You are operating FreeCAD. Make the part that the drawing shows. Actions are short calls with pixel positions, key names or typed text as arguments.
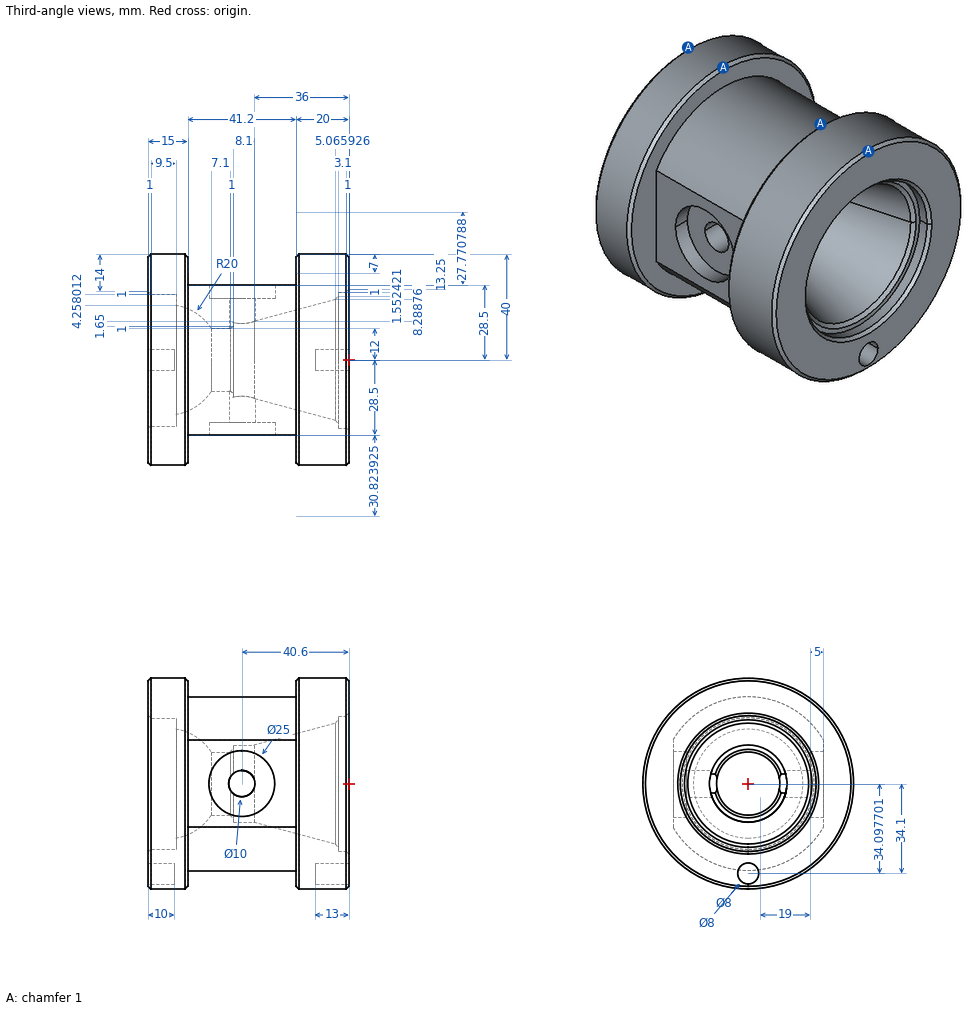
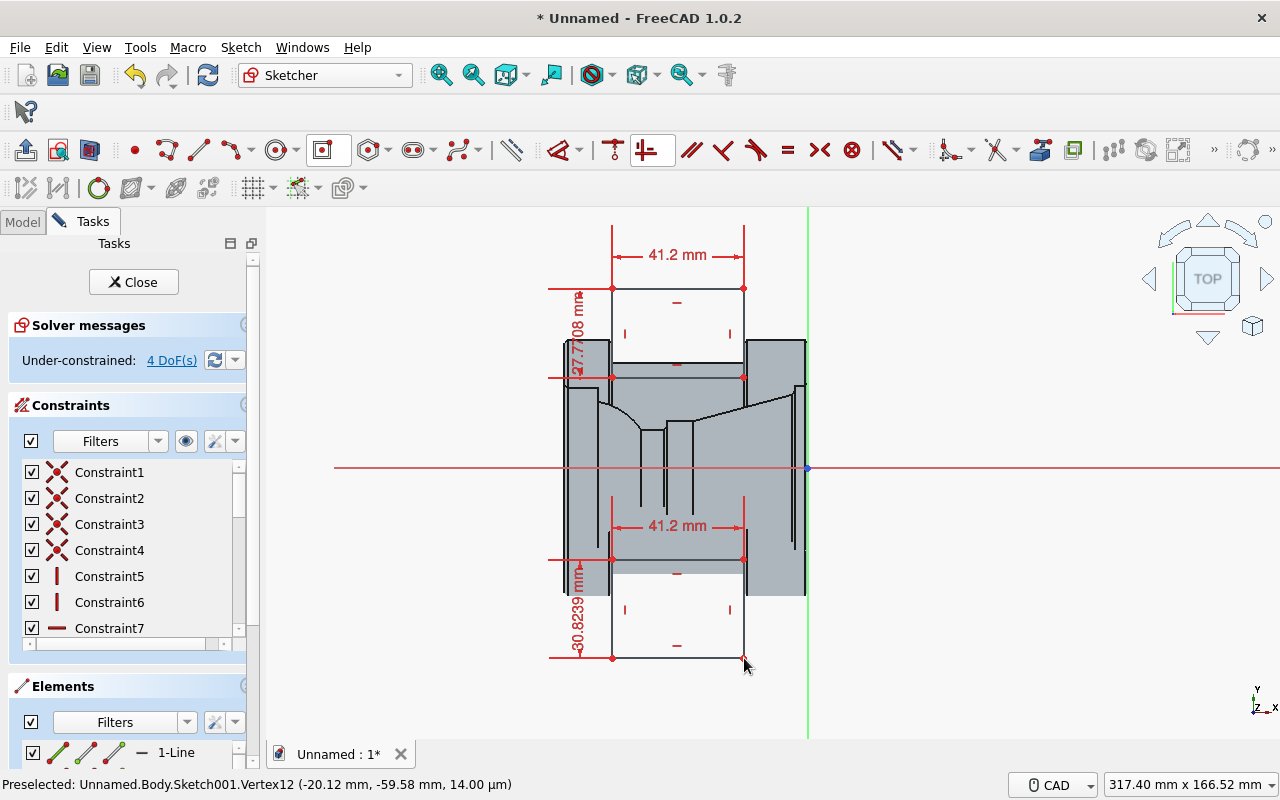
click(558, 150)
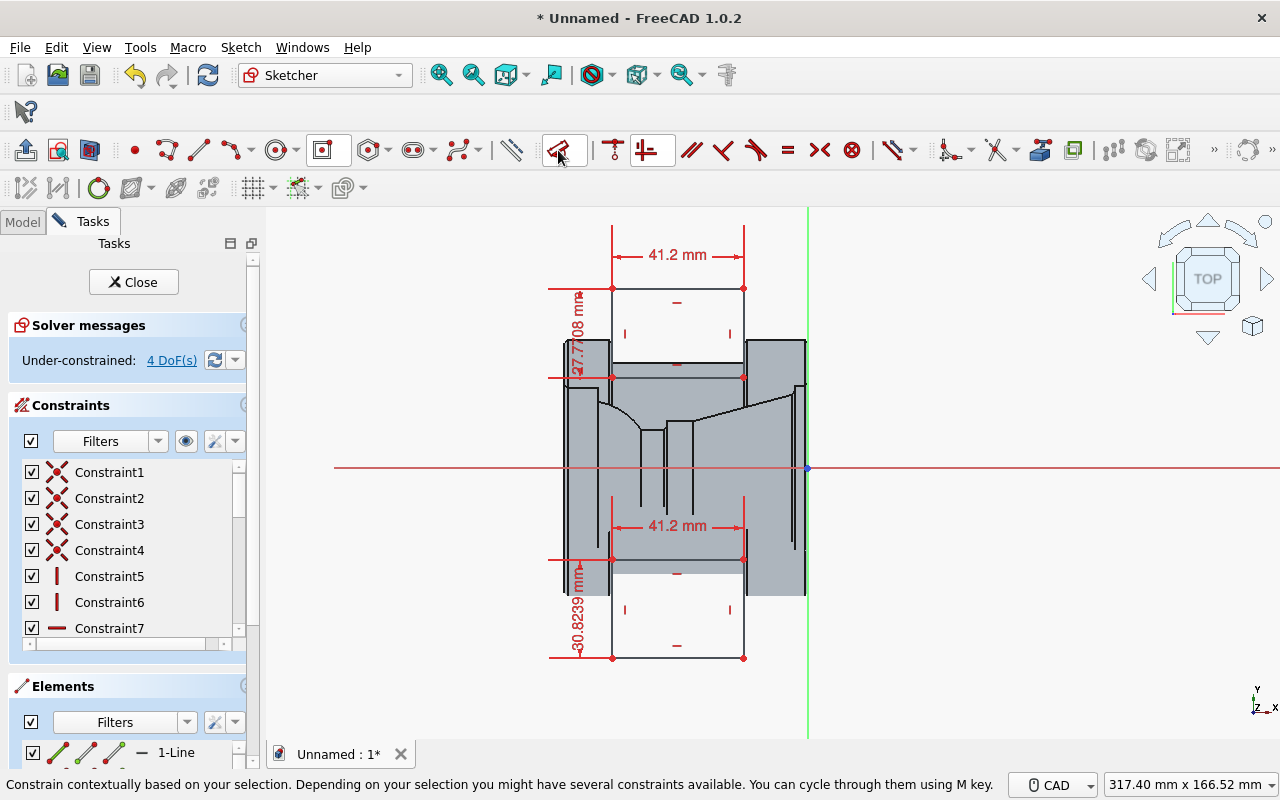
click(744, 378)
click(776, 344)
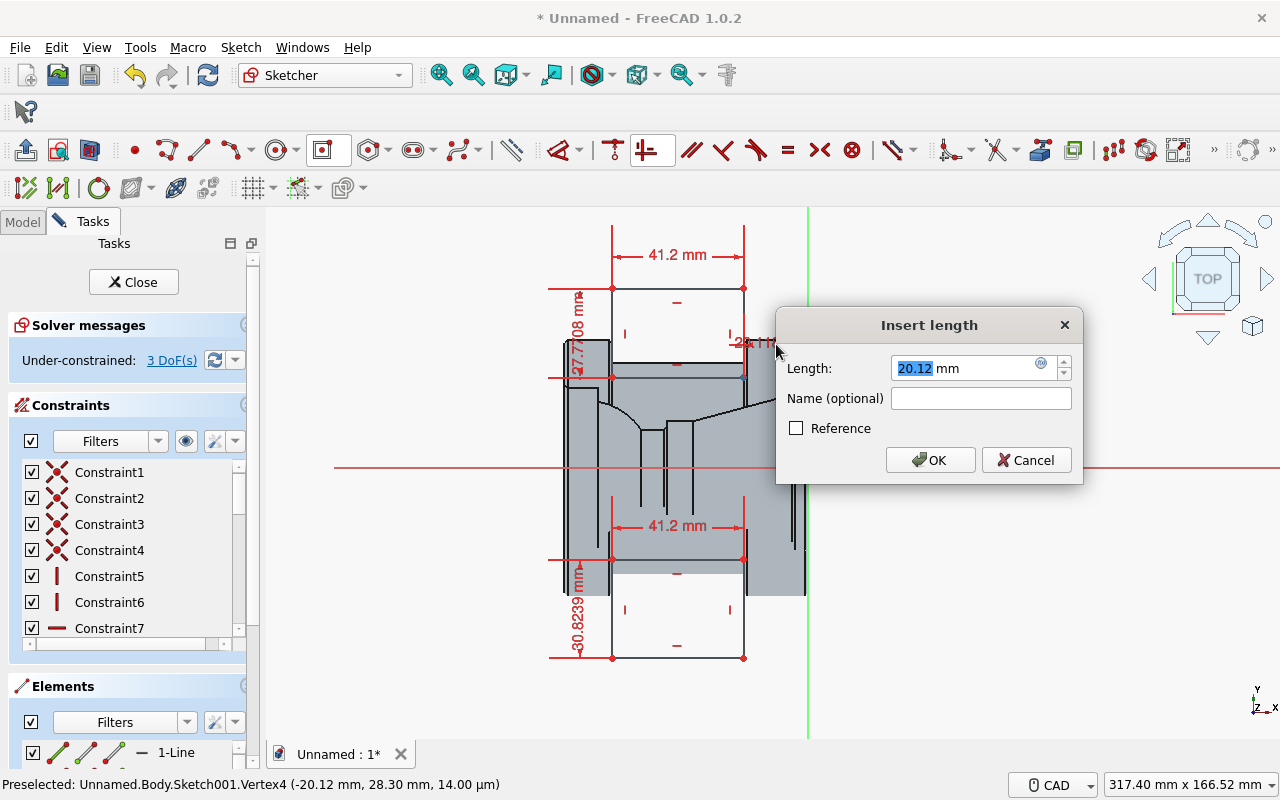
text(20)
key(Return)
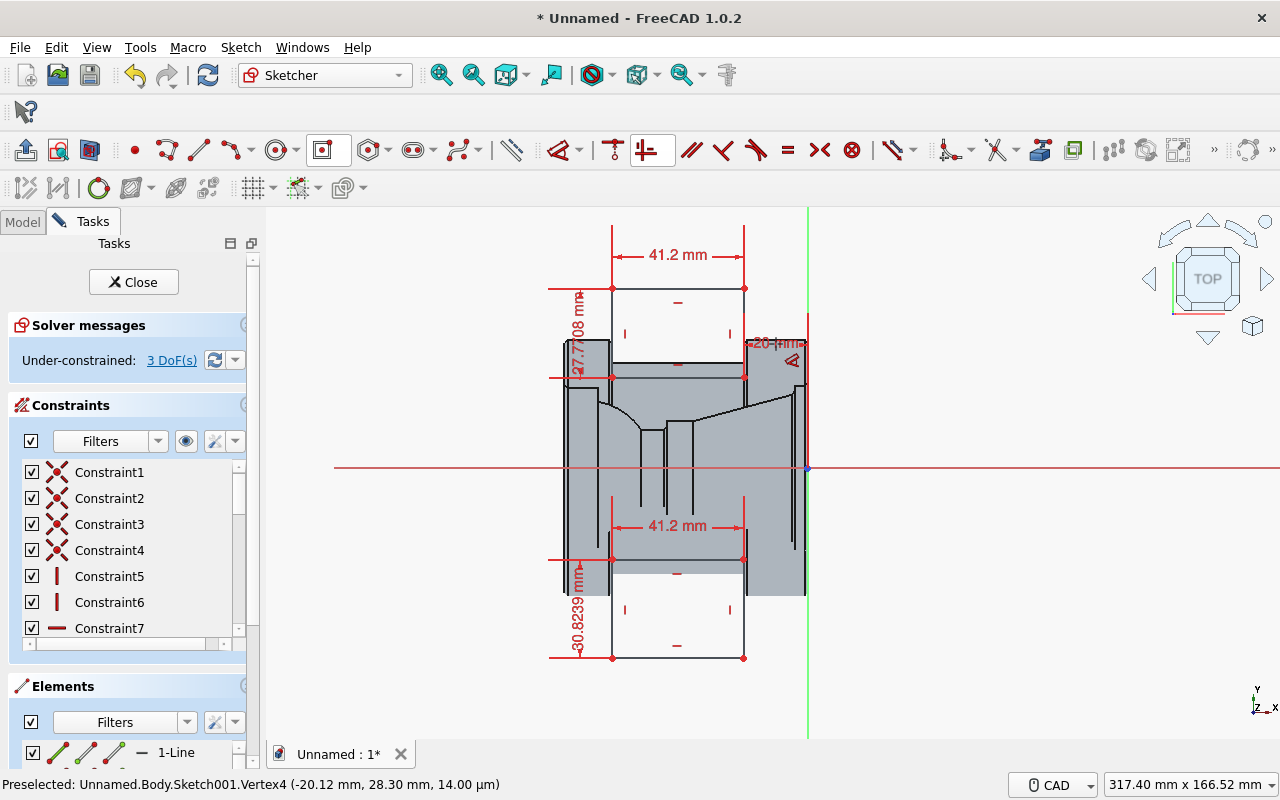
click(744, 658)
click(776, 692)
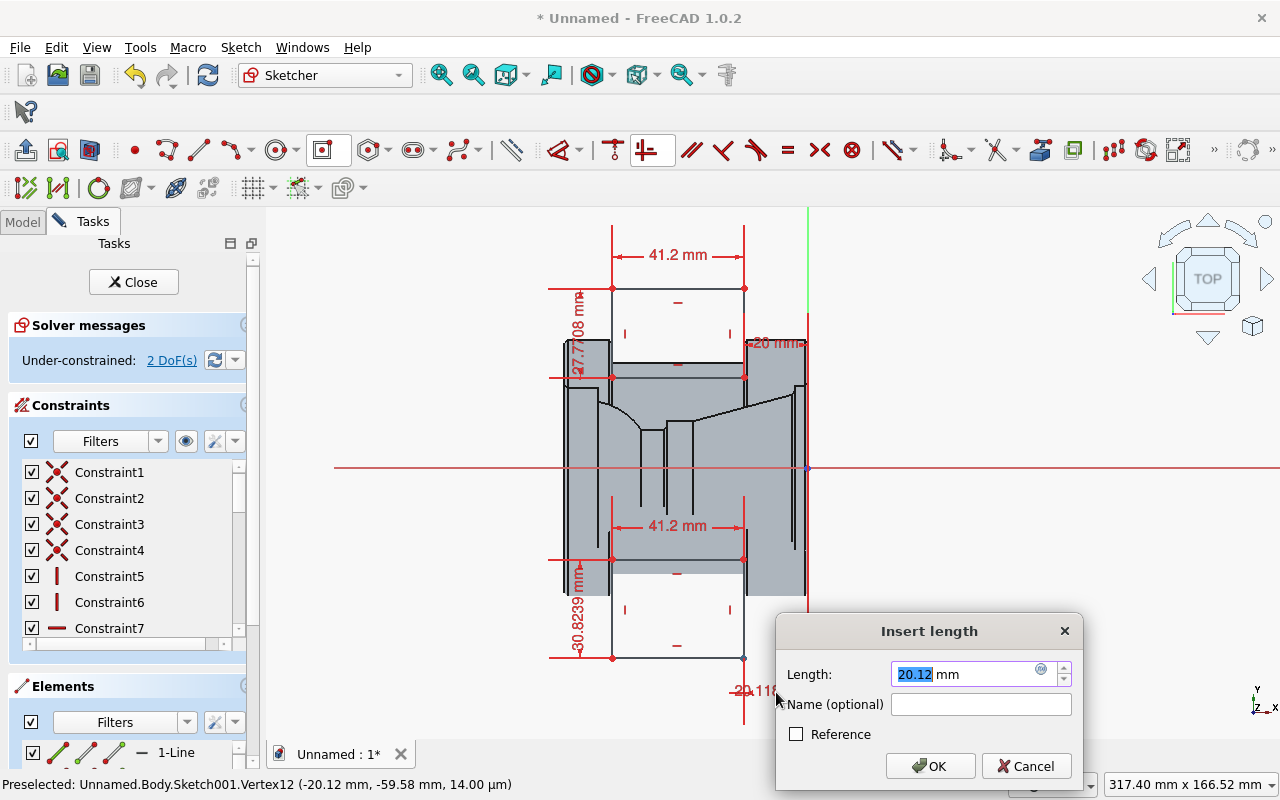
text(20)
key(Return)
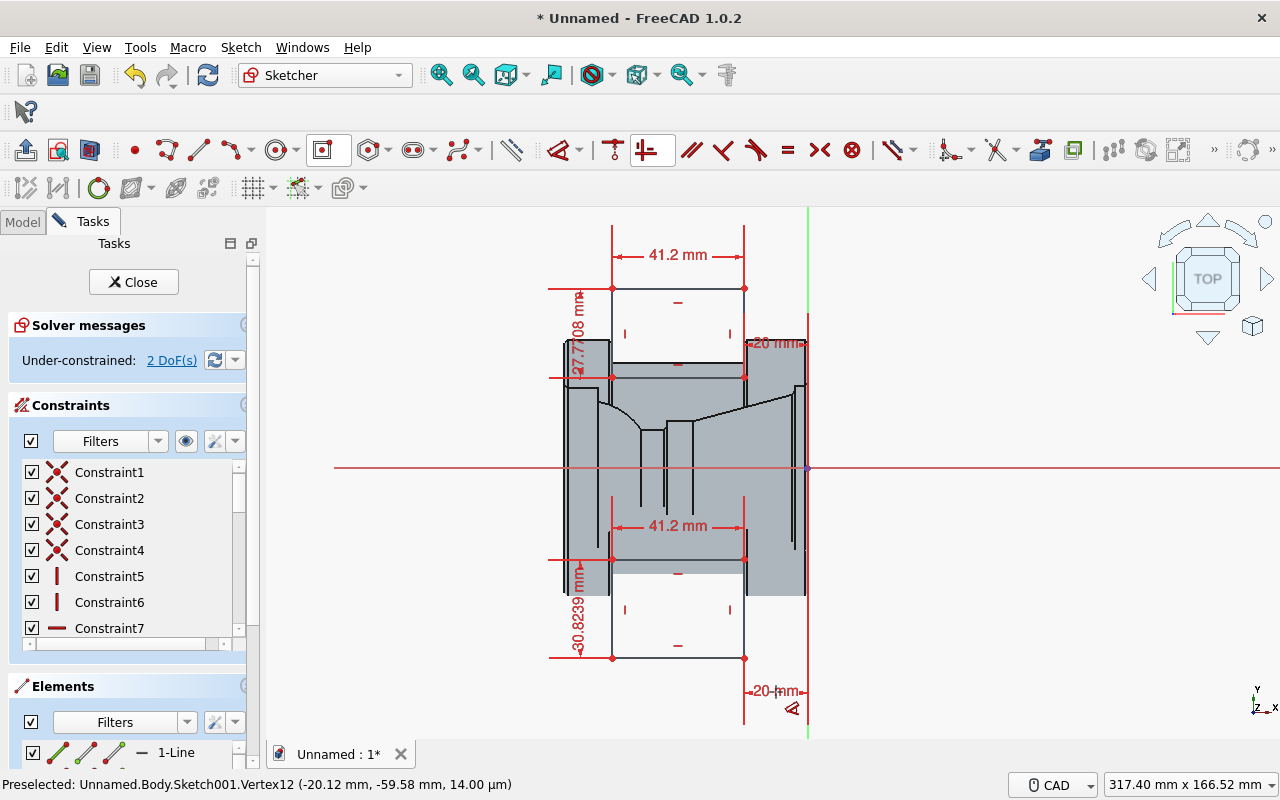
click(612, 378)
click(842, 423)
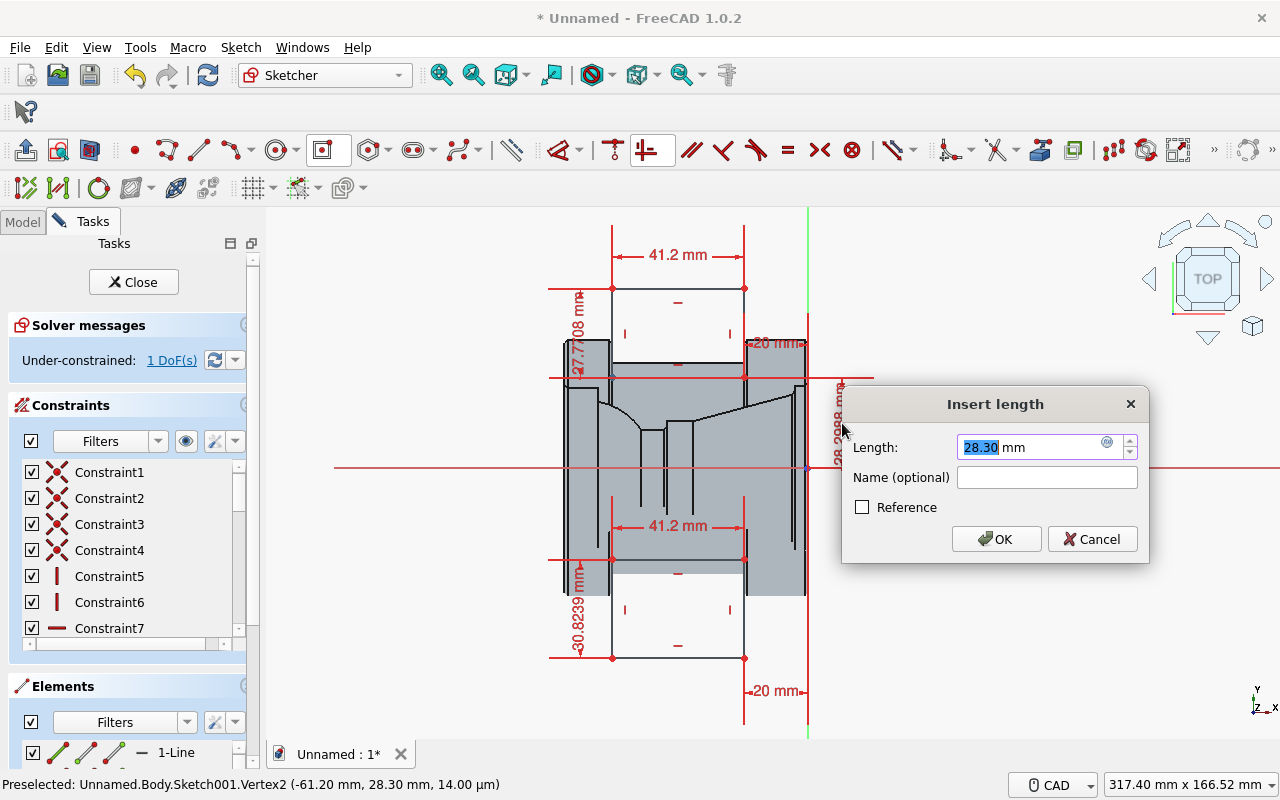
text(28.5)
key(Return)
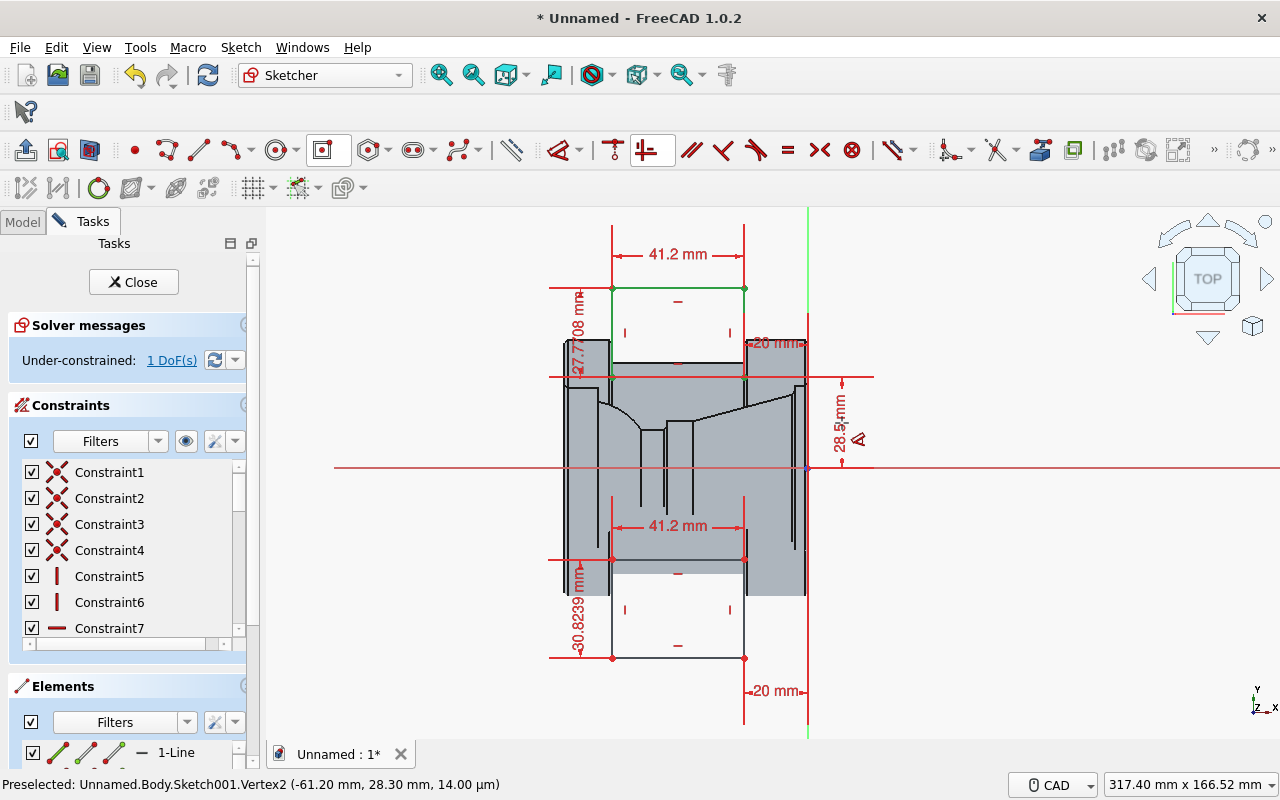
click(612, 560)
click(842, 514)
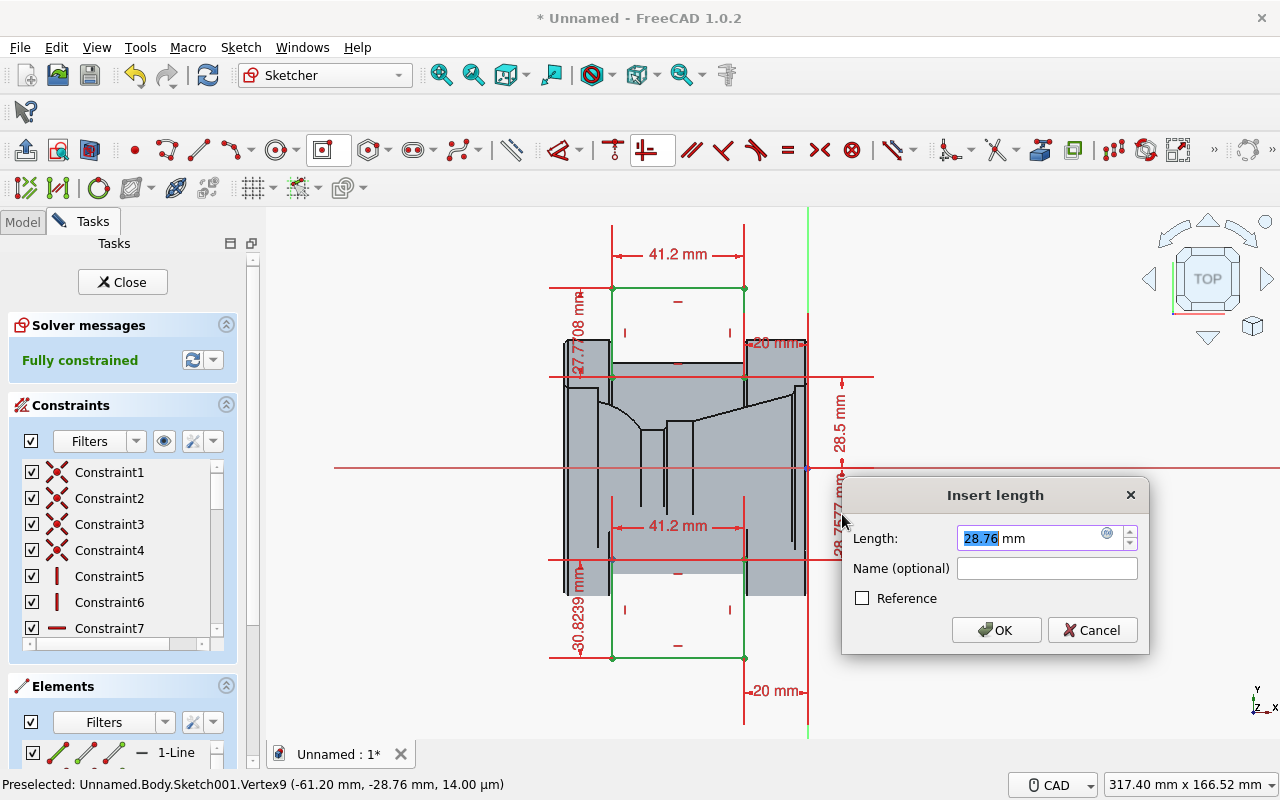
text(28.5)
key(Return)
key(Escape)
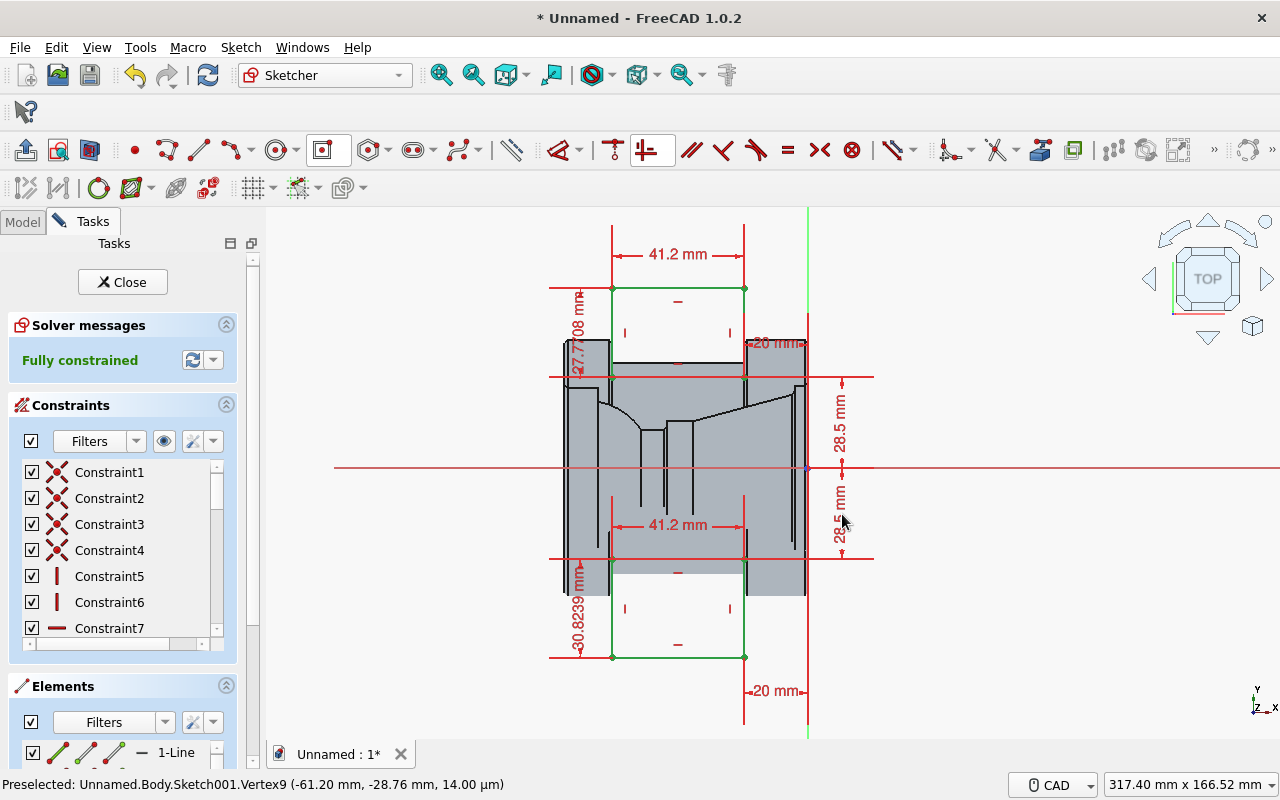
click(123, 282)